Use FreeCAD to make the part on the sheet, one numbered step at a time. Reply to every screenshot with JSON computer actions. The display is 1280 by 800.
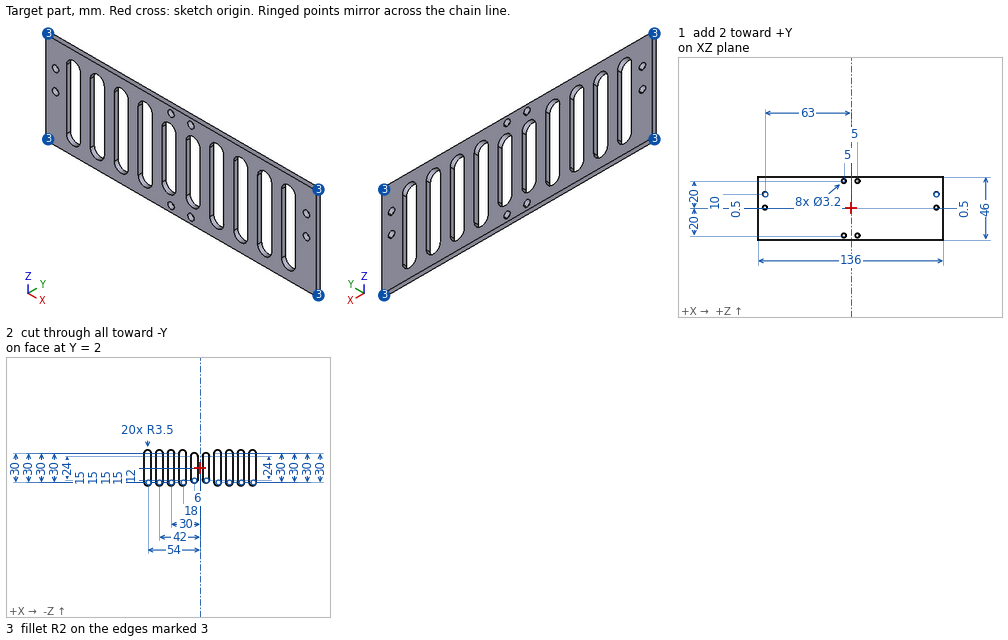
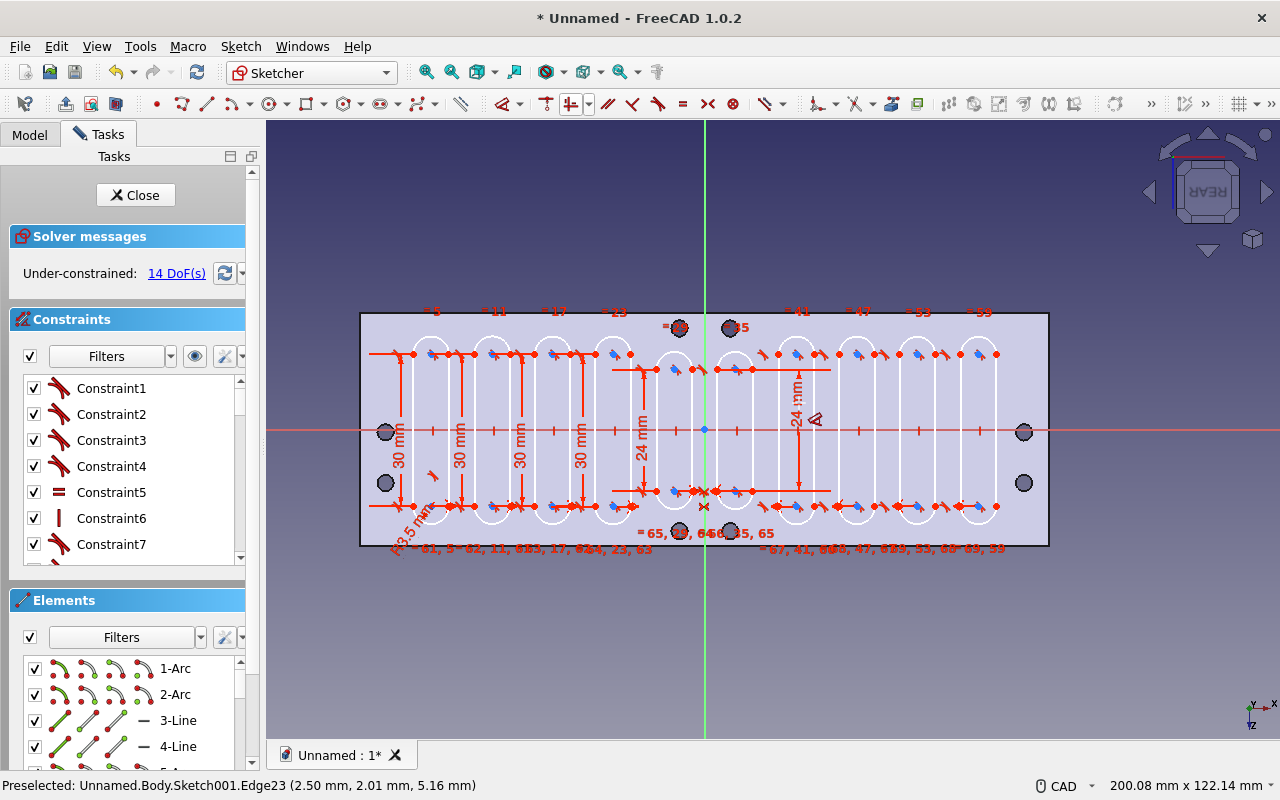
{"action": "left_click", "coordinate": [779, 461]}
{"action": "left_click", "coordinate": [861, 465]}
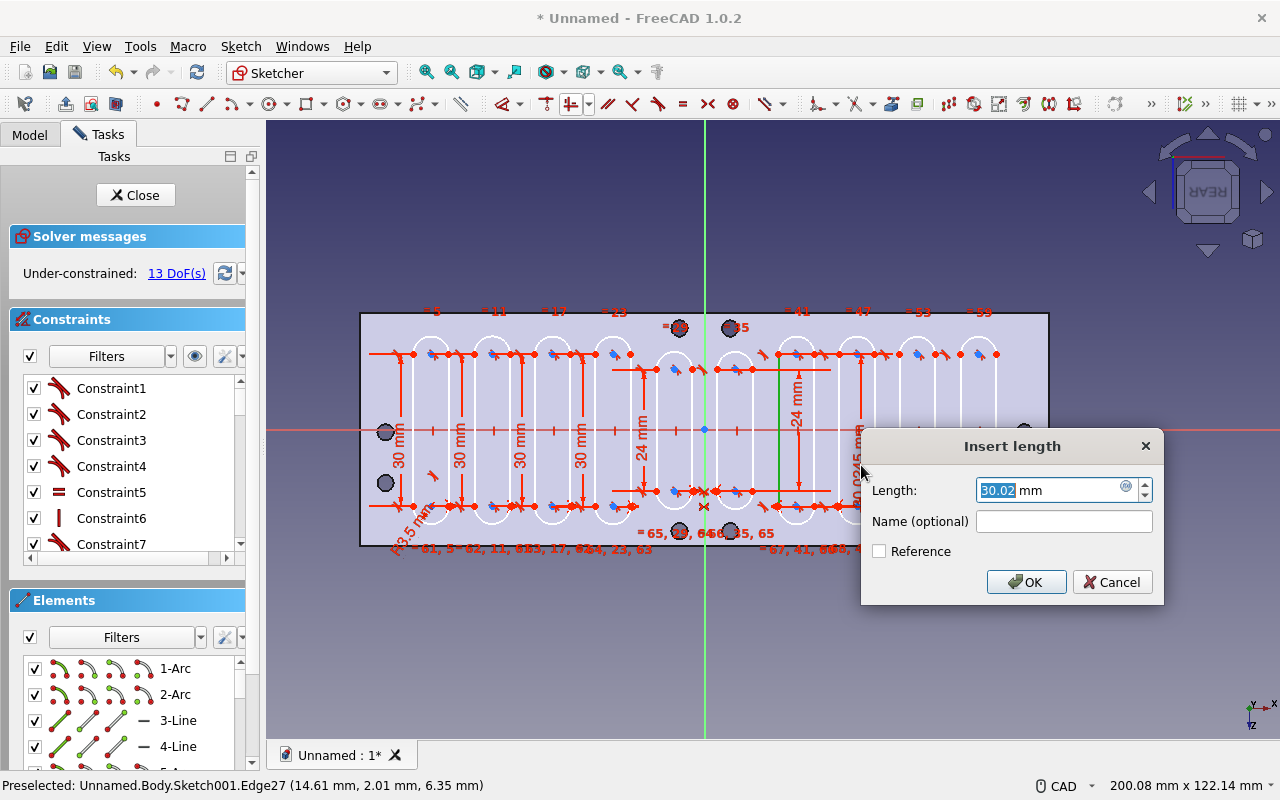
{"action": "type", "text": "30"}
{"action": "key", "text": "Return"}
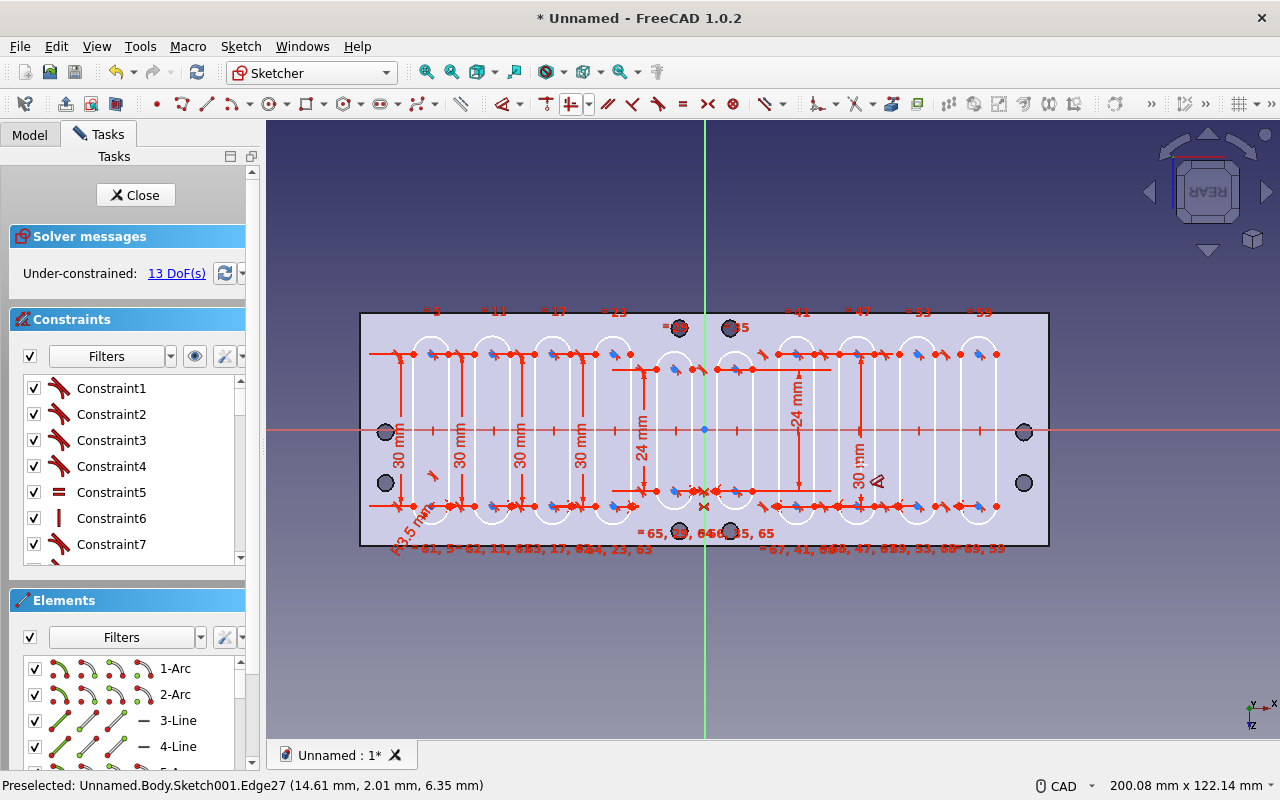
{"action": "left_click", "coordinate": [839, 461]}
{"action": "left_click", "coordinate": [921, 395]}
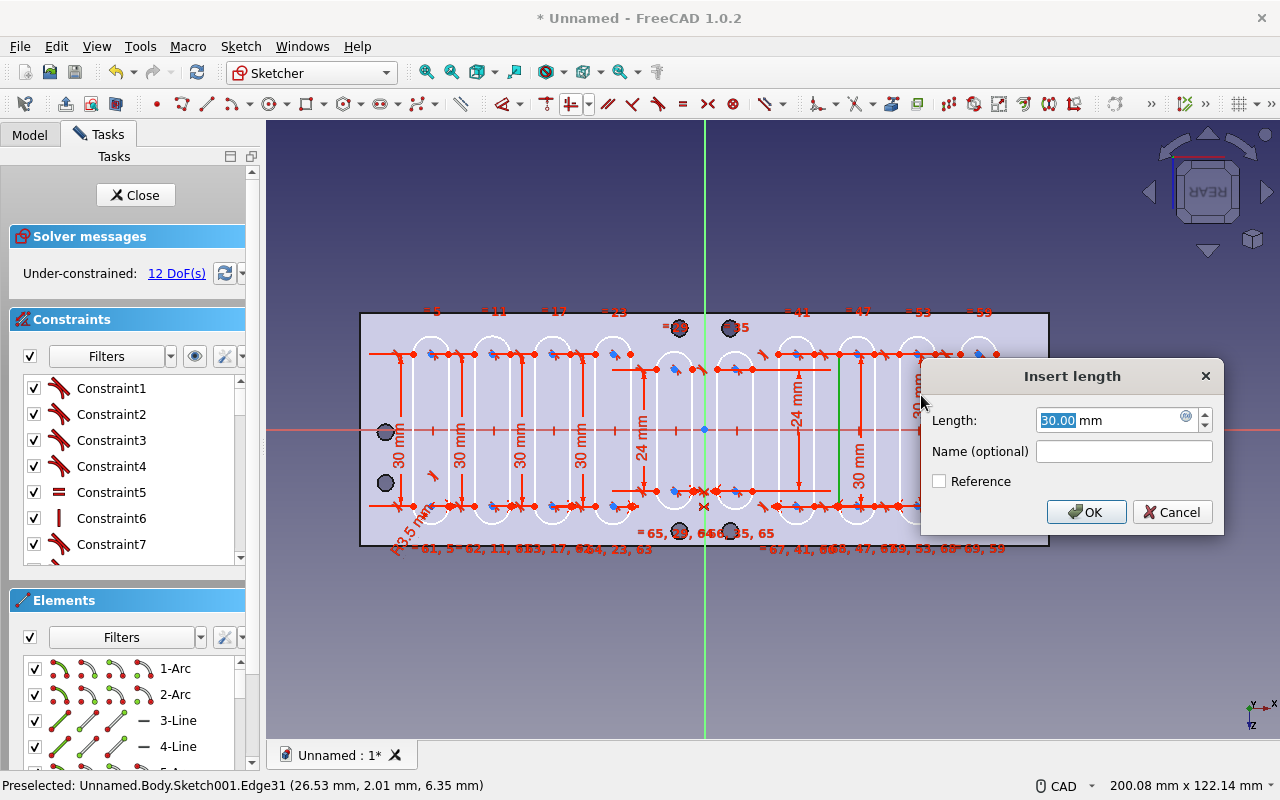
{"action": "type", "text": "30"}
{"action": "key", "text": "Return"}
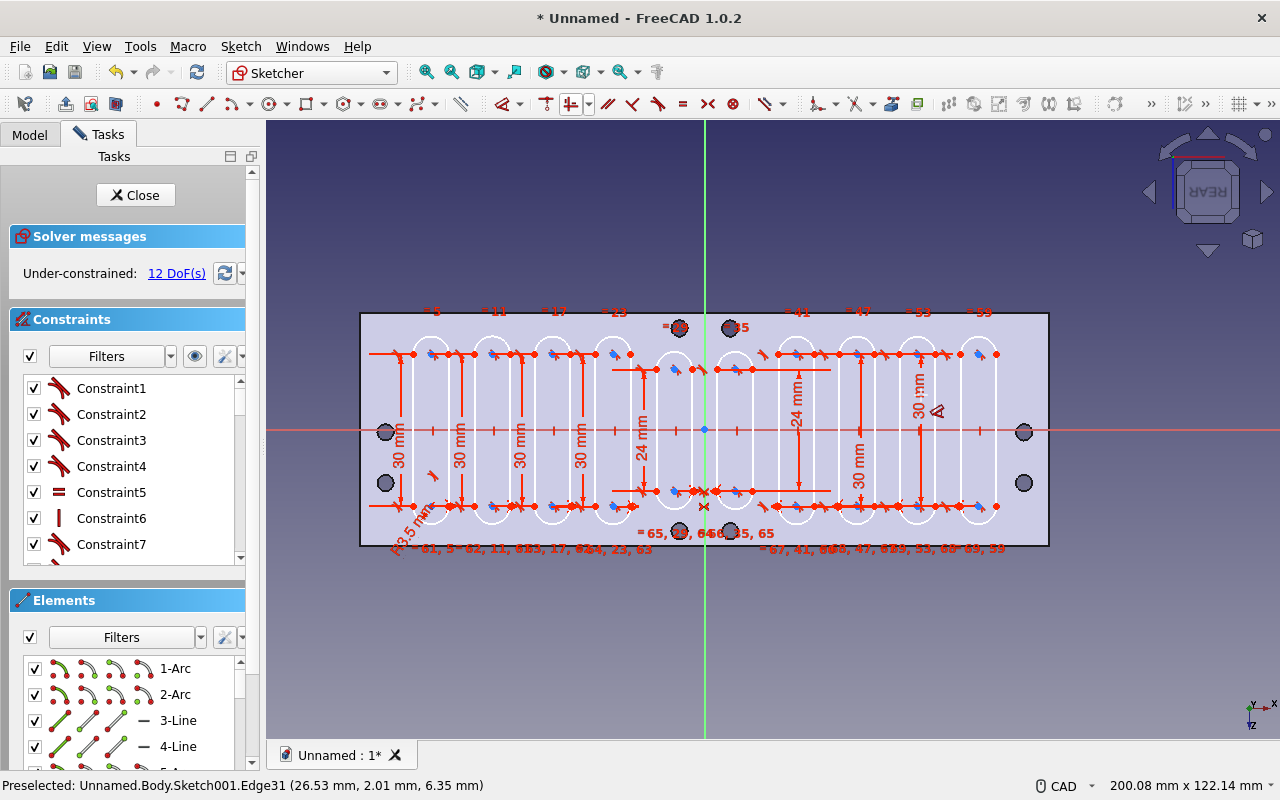
{"action": "left_click", "coordinate": [900, 461]}
{"action": "left_click", "coordinate": [982, 465]}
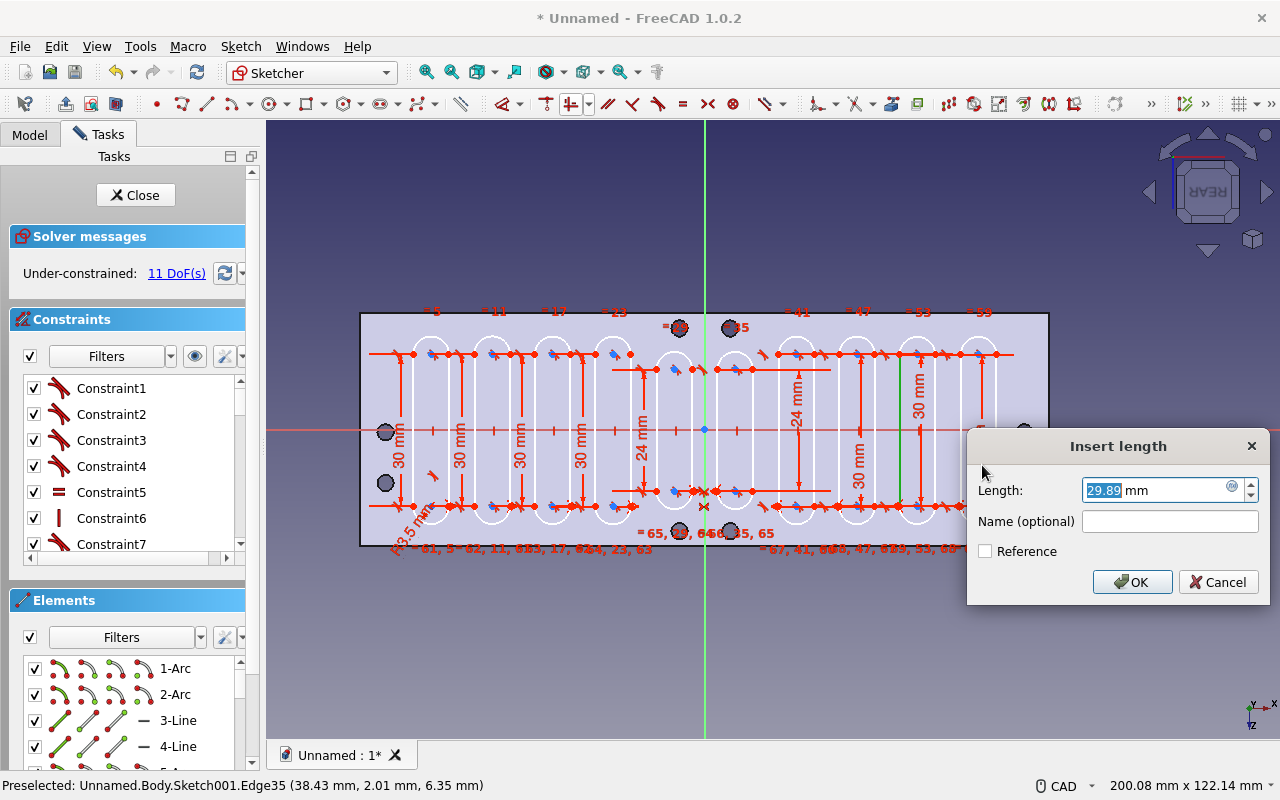
{"action": "type", "text": "30"}
{"action": "key", "text": "Return"}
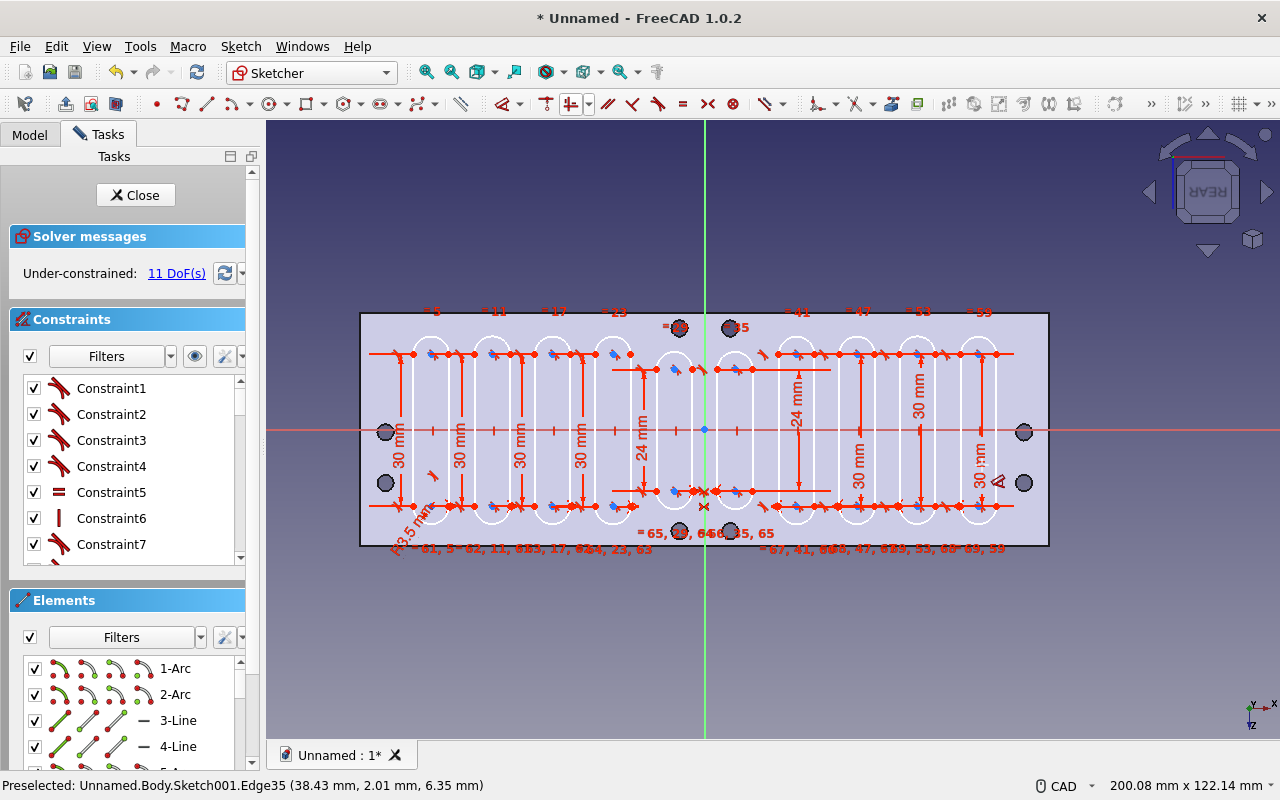
{"action": "left_click", "coordinate": [961, 461]}
{"action": "left_click", "coordinate": [1019, 396]}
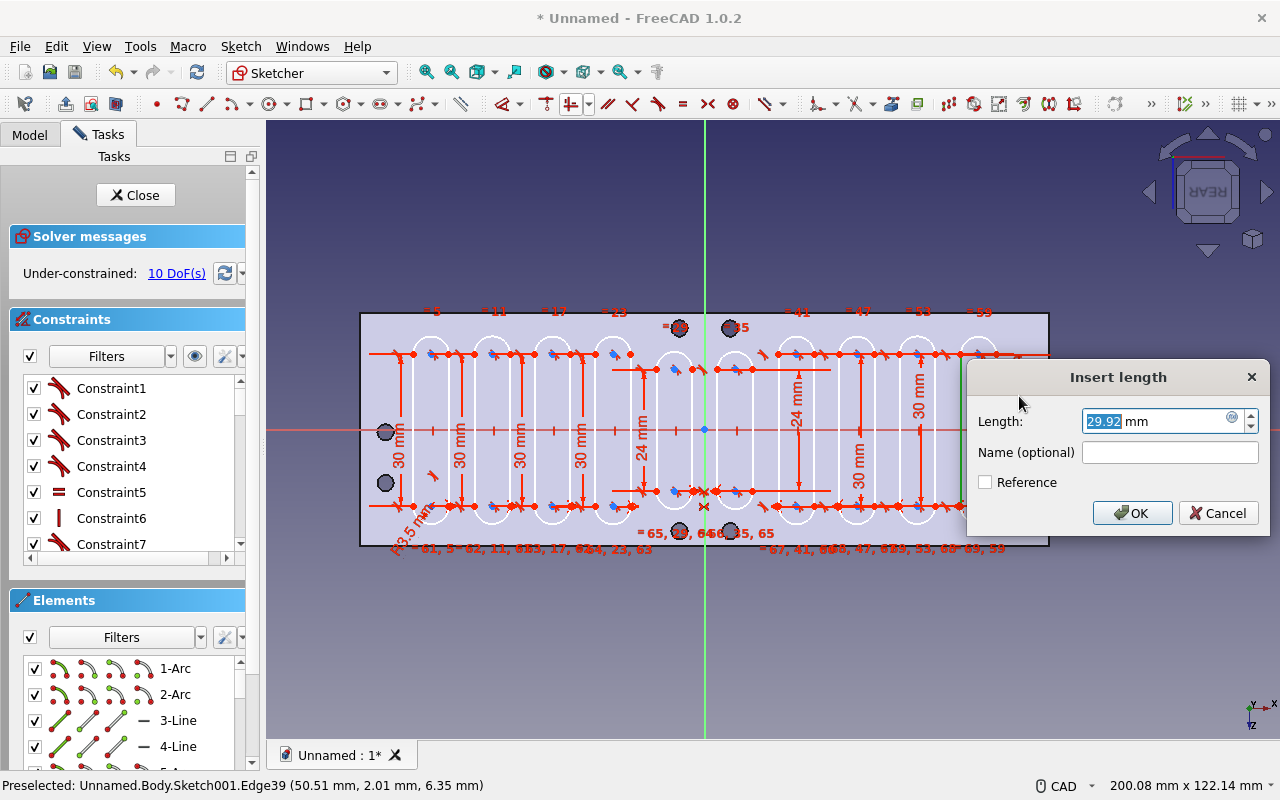
{"action": "type", "text": "30"}
{"action": "key", "text": "Return"}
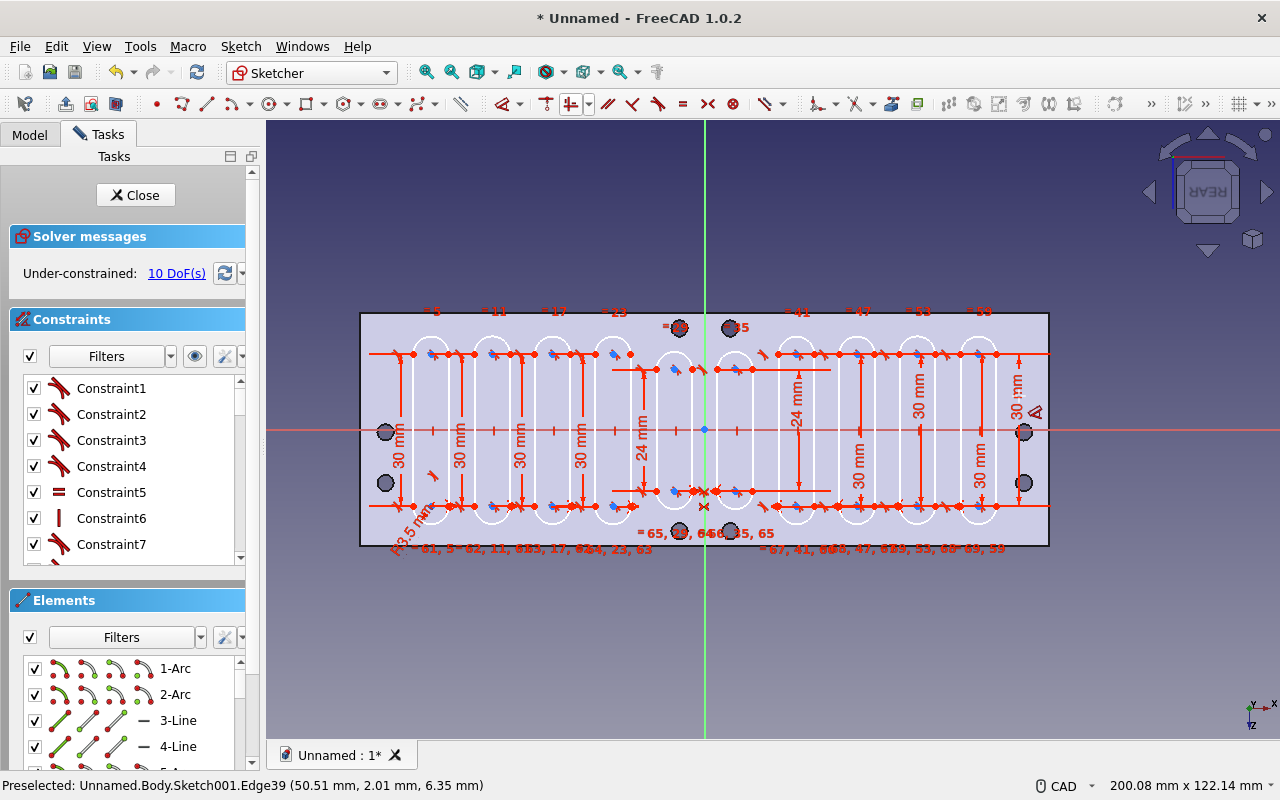
{"action": "scroll", "coordinate": [674, 491], "scroll_direction": "up", "scroll_amount": 2}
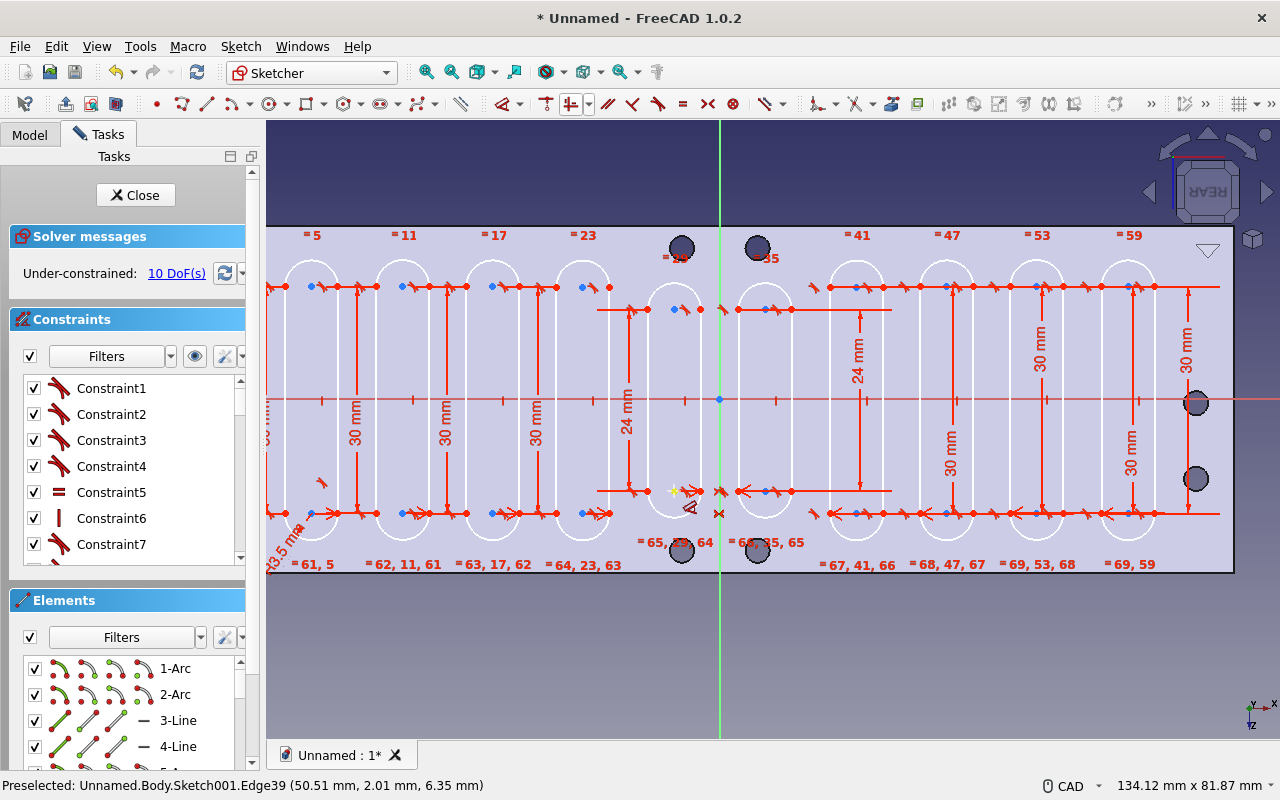
{"action": "left_click", "coordinate": [674, 491]}
{"action": "left_click", "coordinate": [697, 525]}